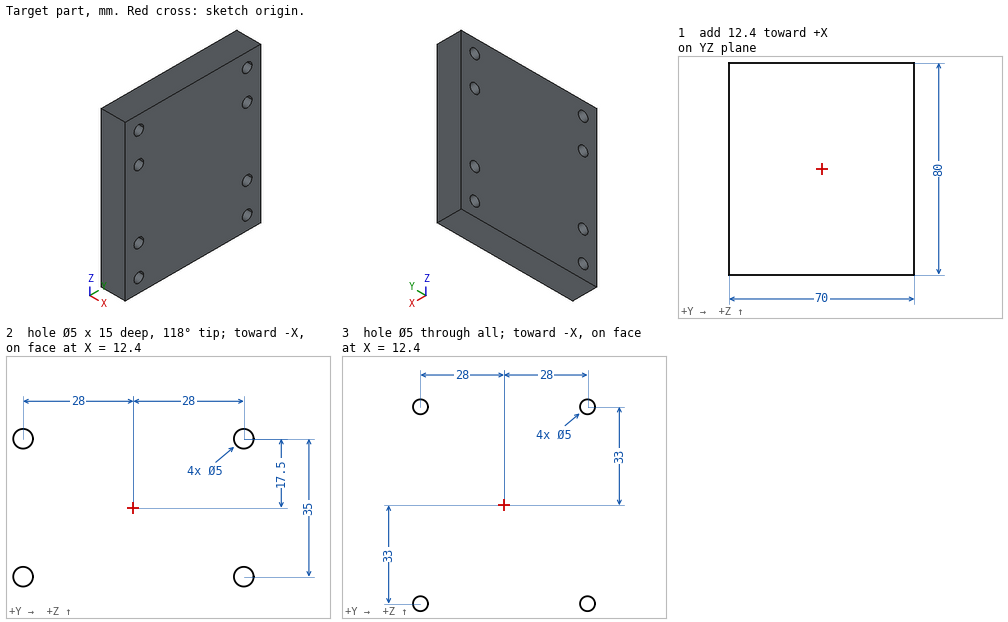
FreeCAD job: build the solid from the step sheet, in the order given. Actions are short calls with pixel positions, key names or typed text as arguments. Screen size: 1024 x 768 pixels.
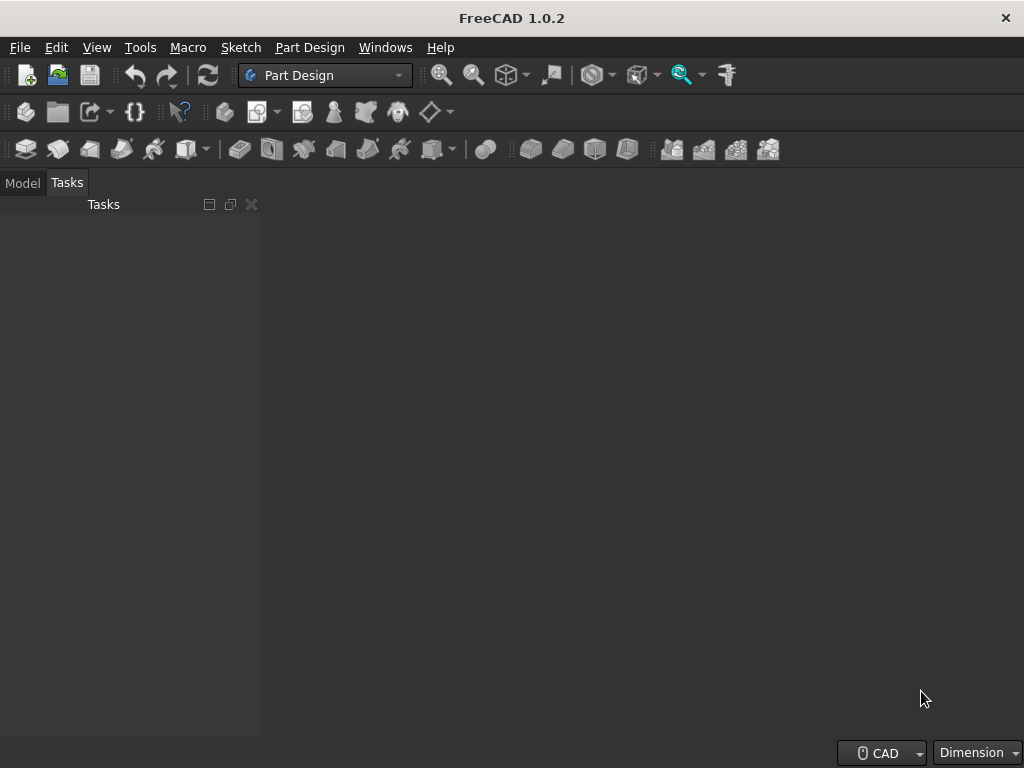
click(542, 76)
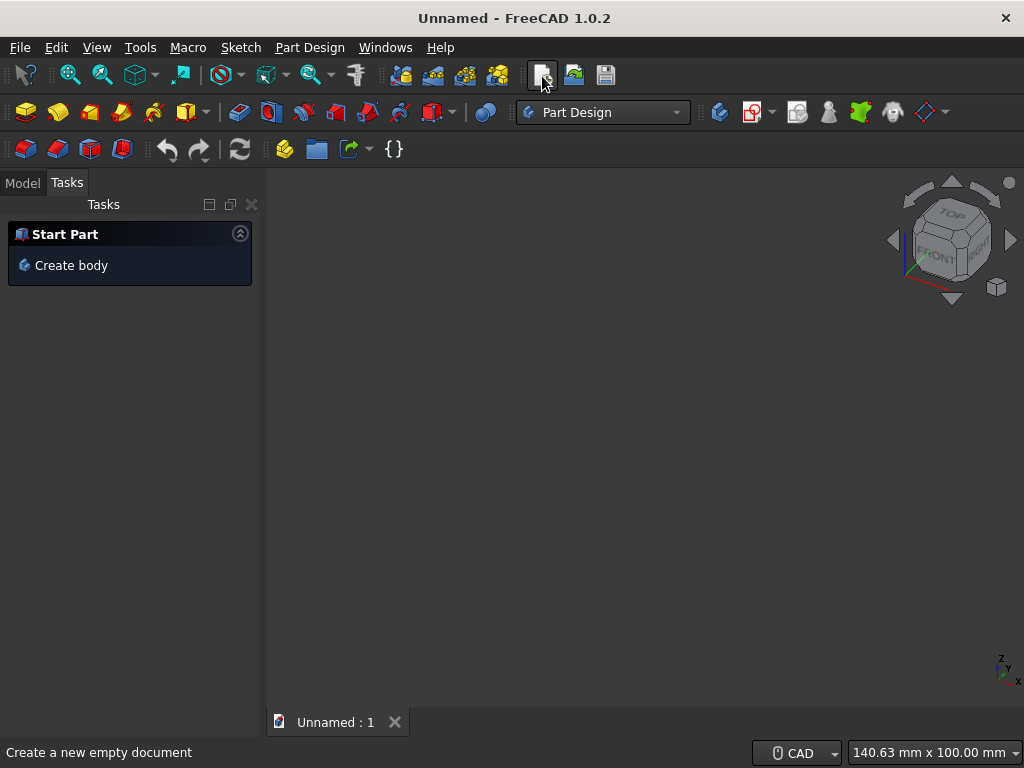
click(752, 112)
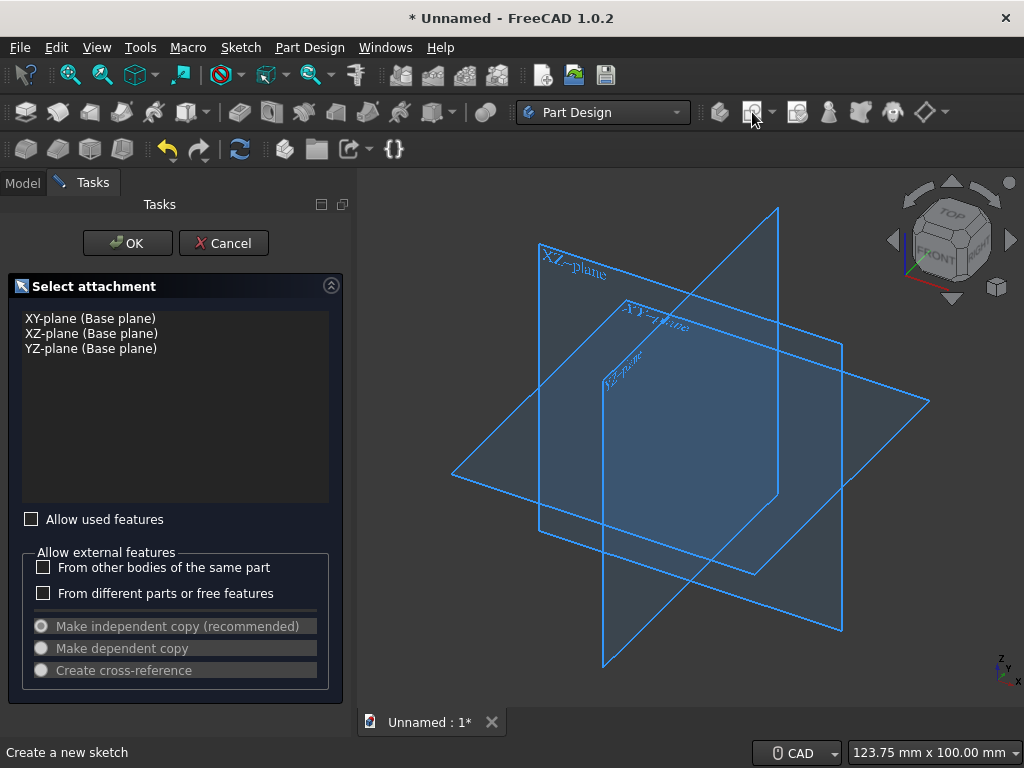
click(82, 348)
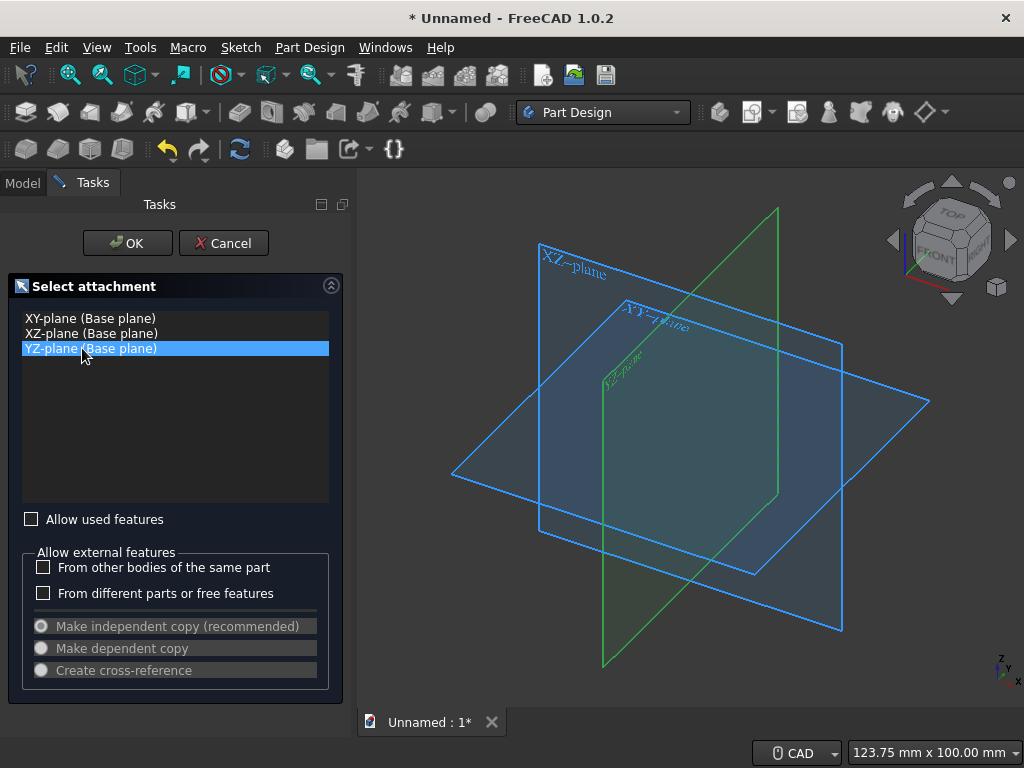
click(128, 243)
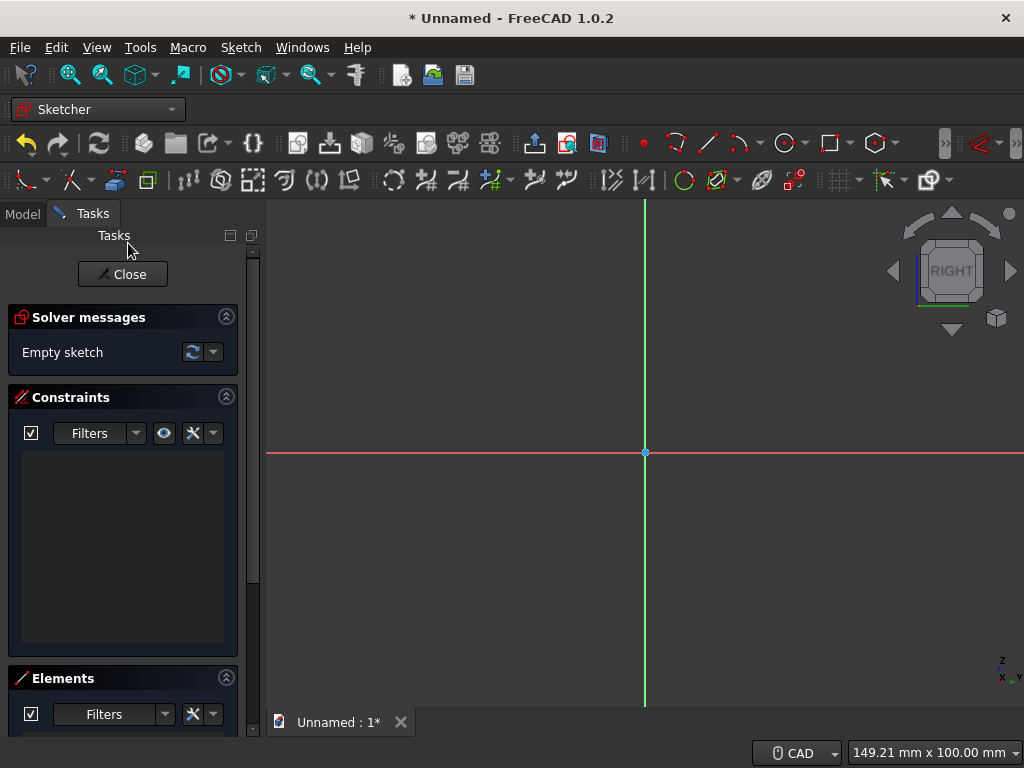
scroll(294, 453, down, 1)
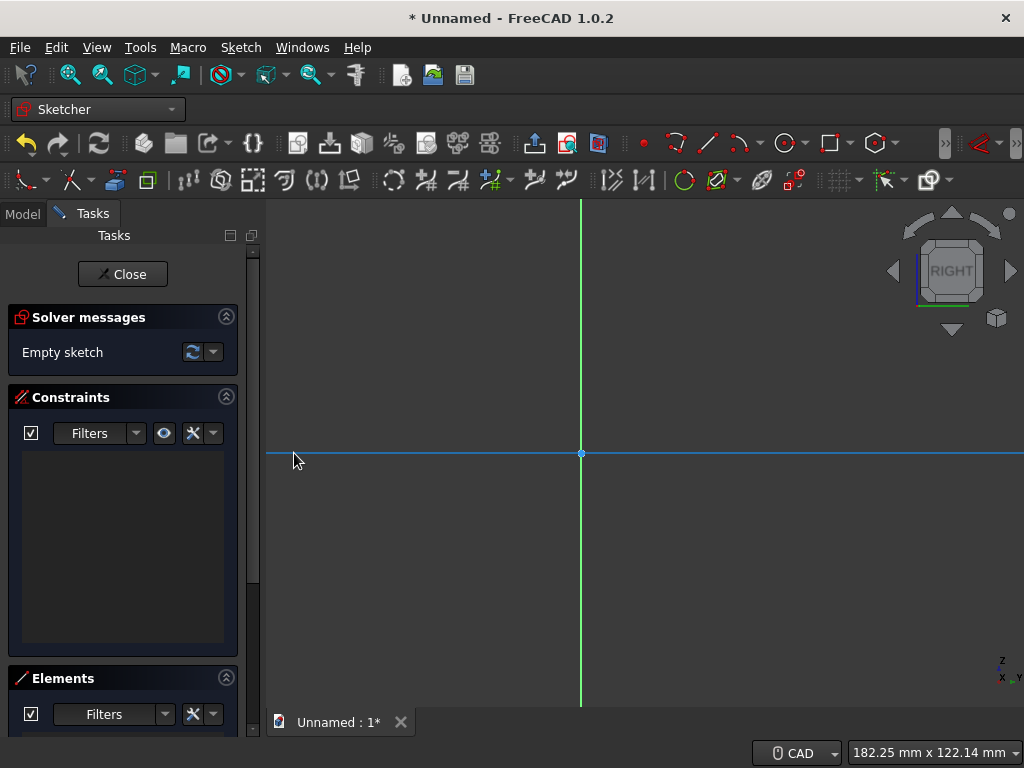
key(g)
key(v)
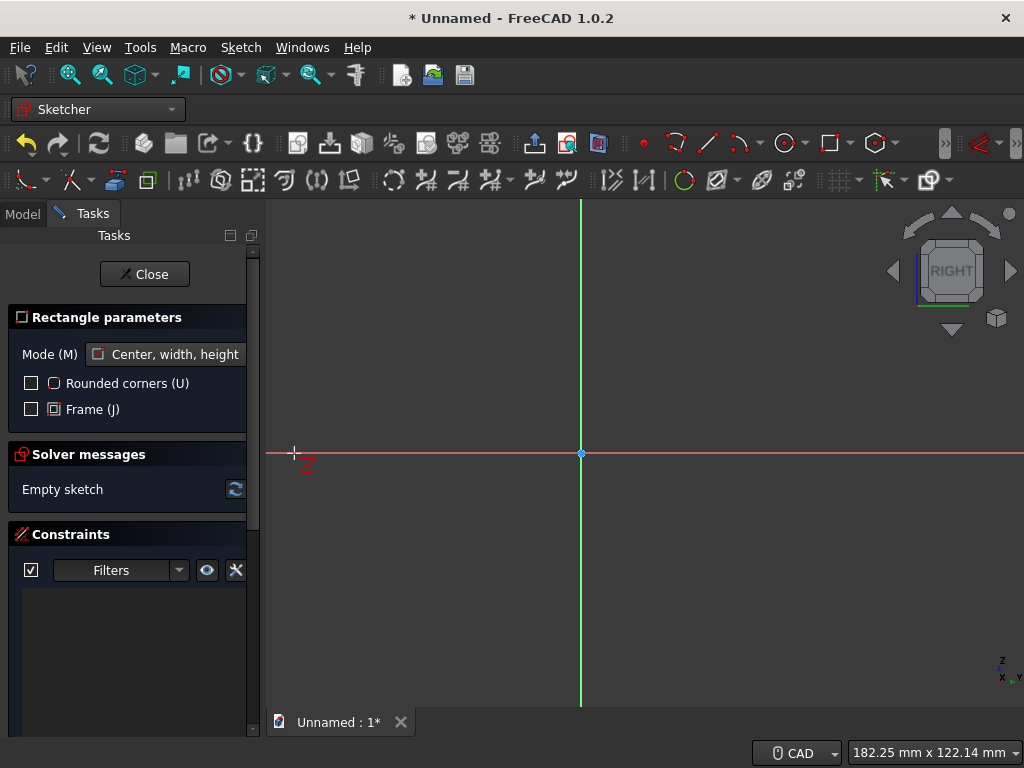
click(581, 453)
move(727, 287)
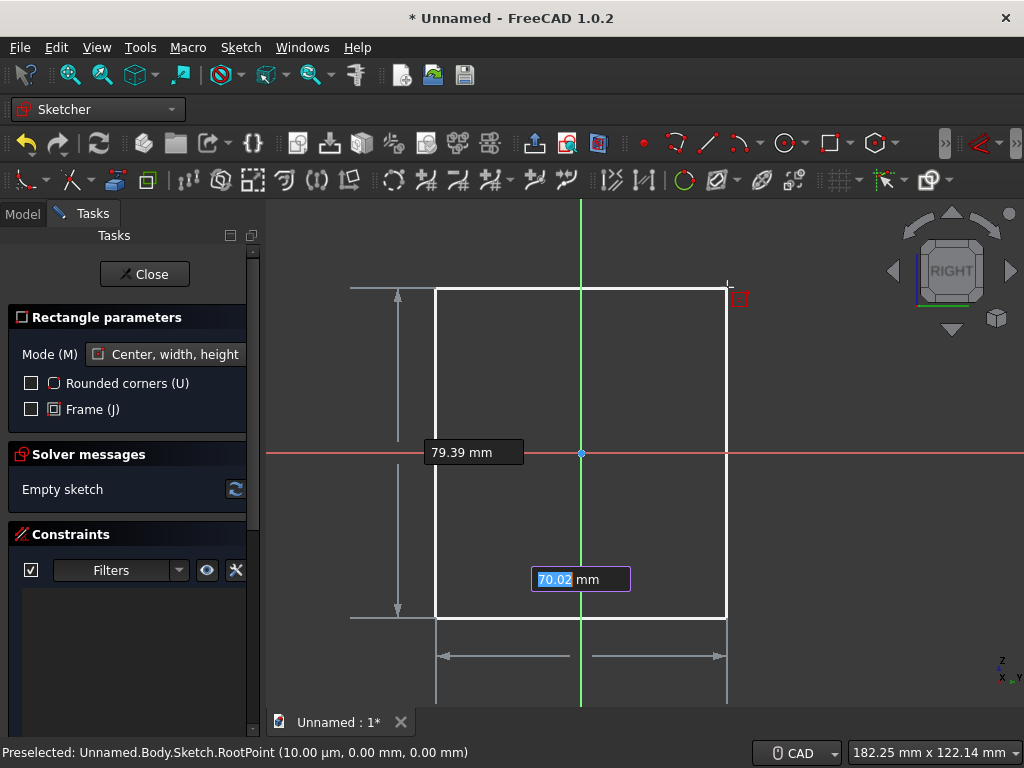
text(70)
key(Tab)
text(80)
key(Return)
key(Escape)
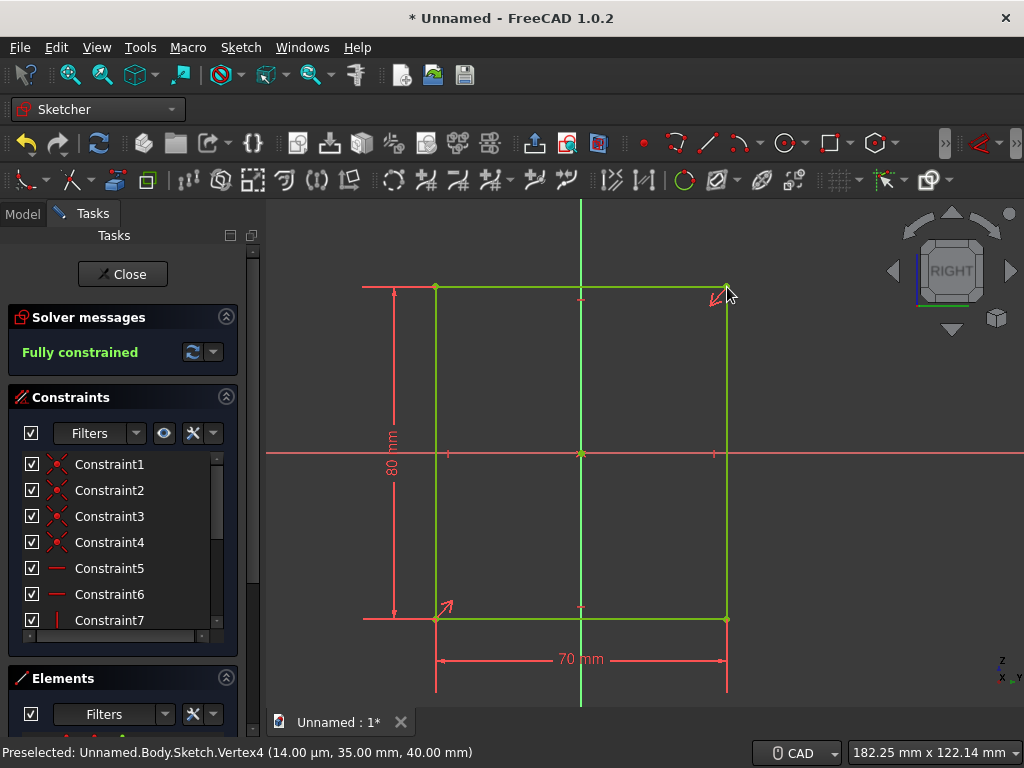
click(123, 274)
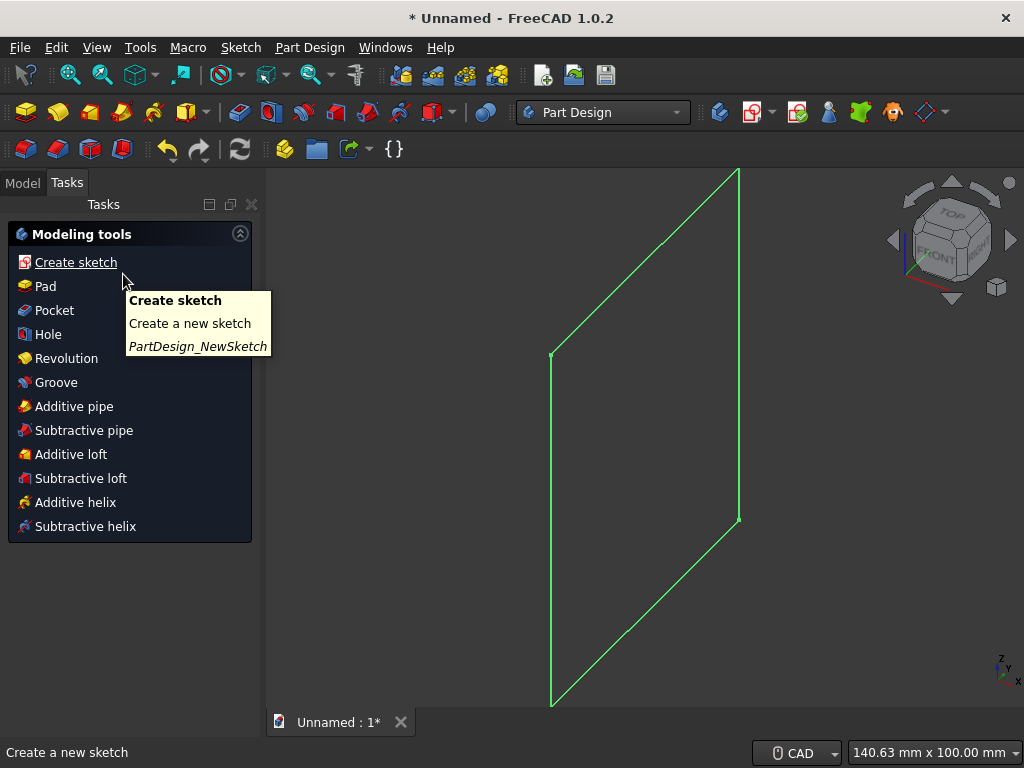
click(26, 112)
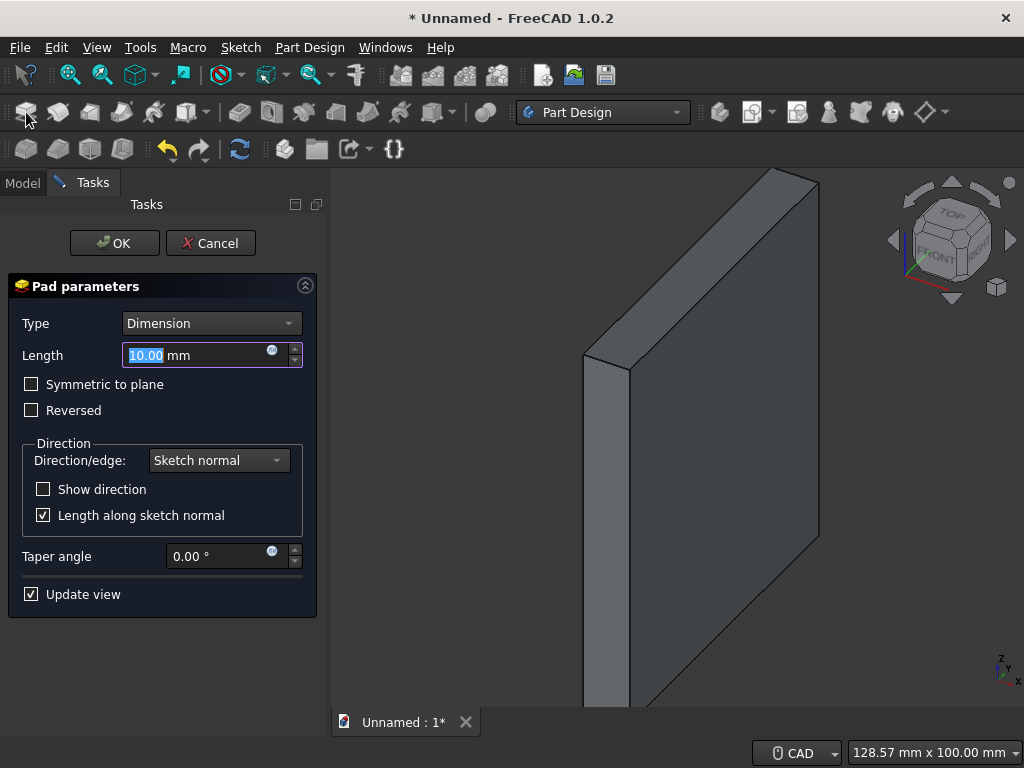
text(12.4)
key(Tab)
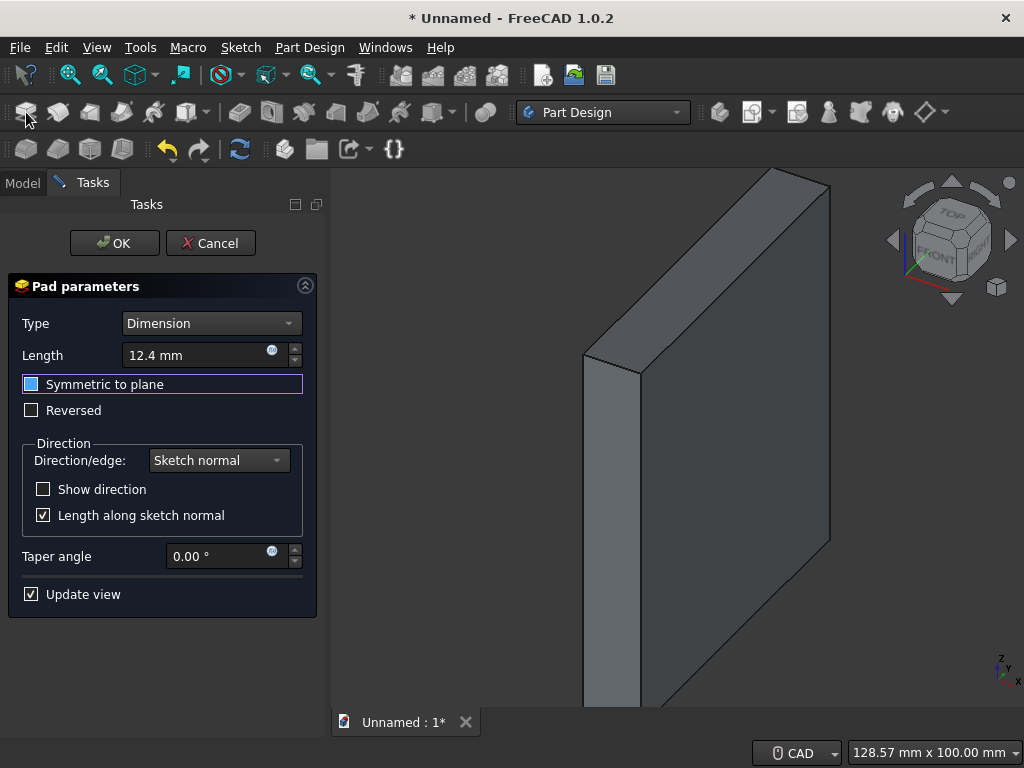
click(115, 243)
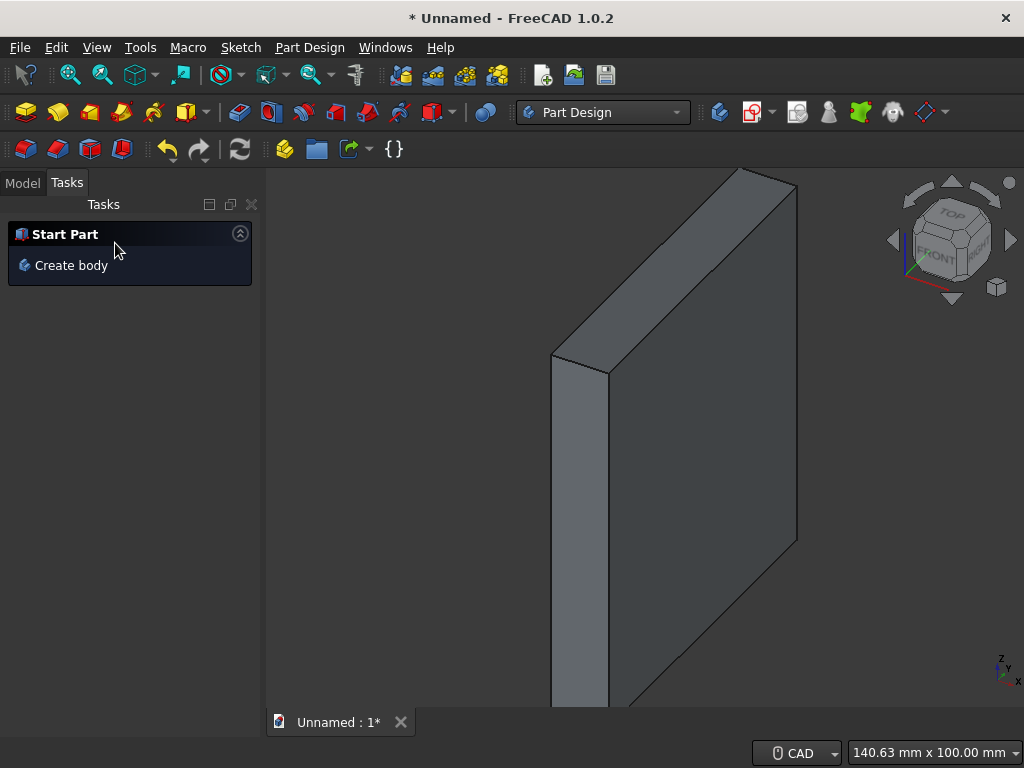
click(72, 76)